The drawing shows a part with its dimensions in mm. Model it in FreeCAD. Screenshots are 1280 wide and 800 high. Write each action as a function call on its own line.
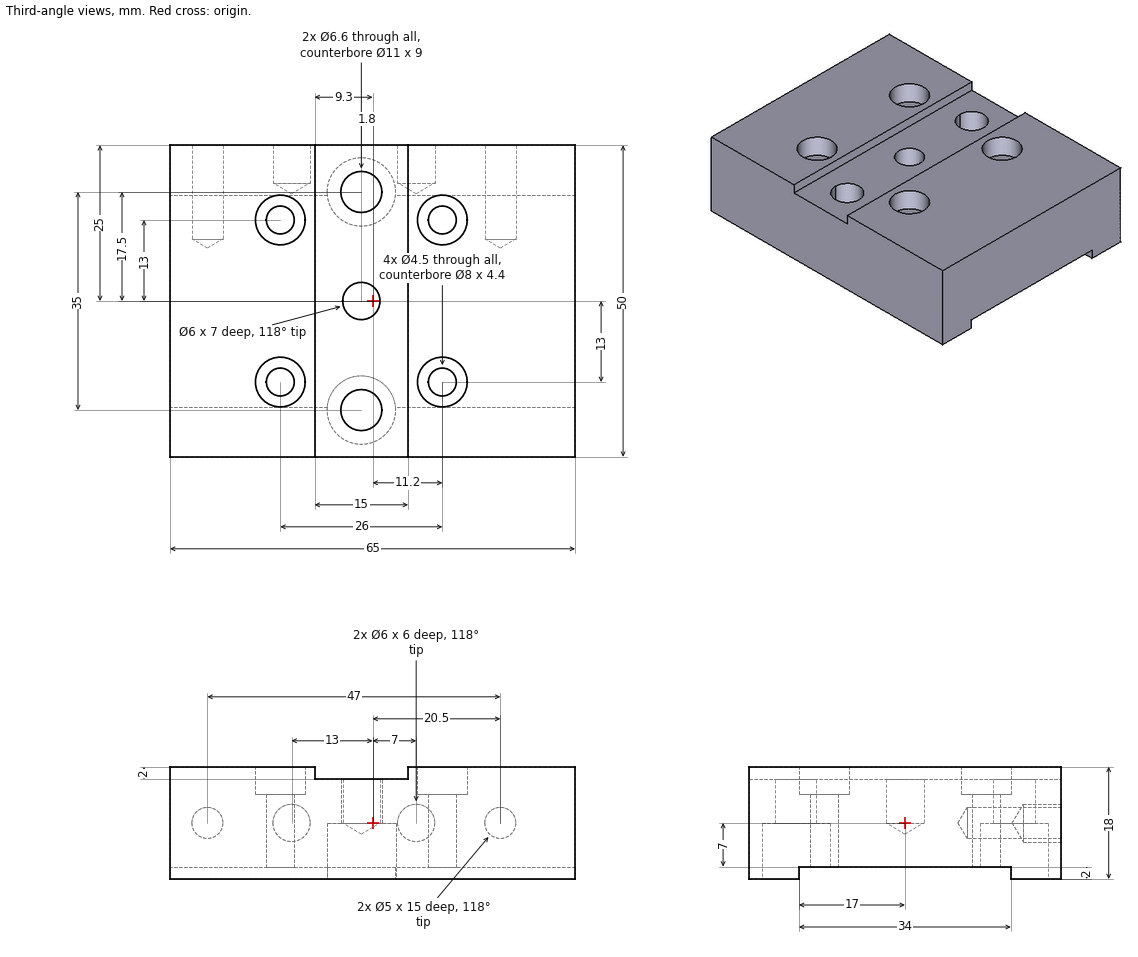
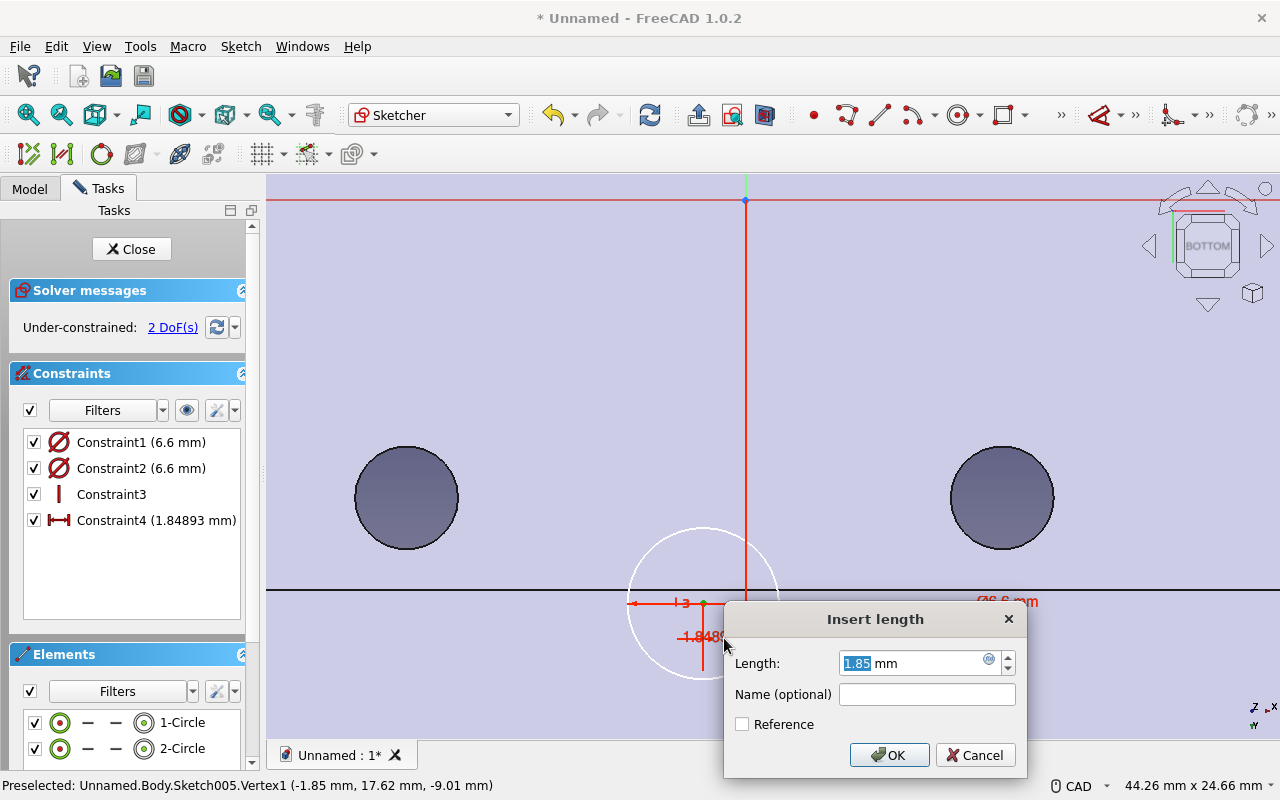
text(1.8)
key(Return)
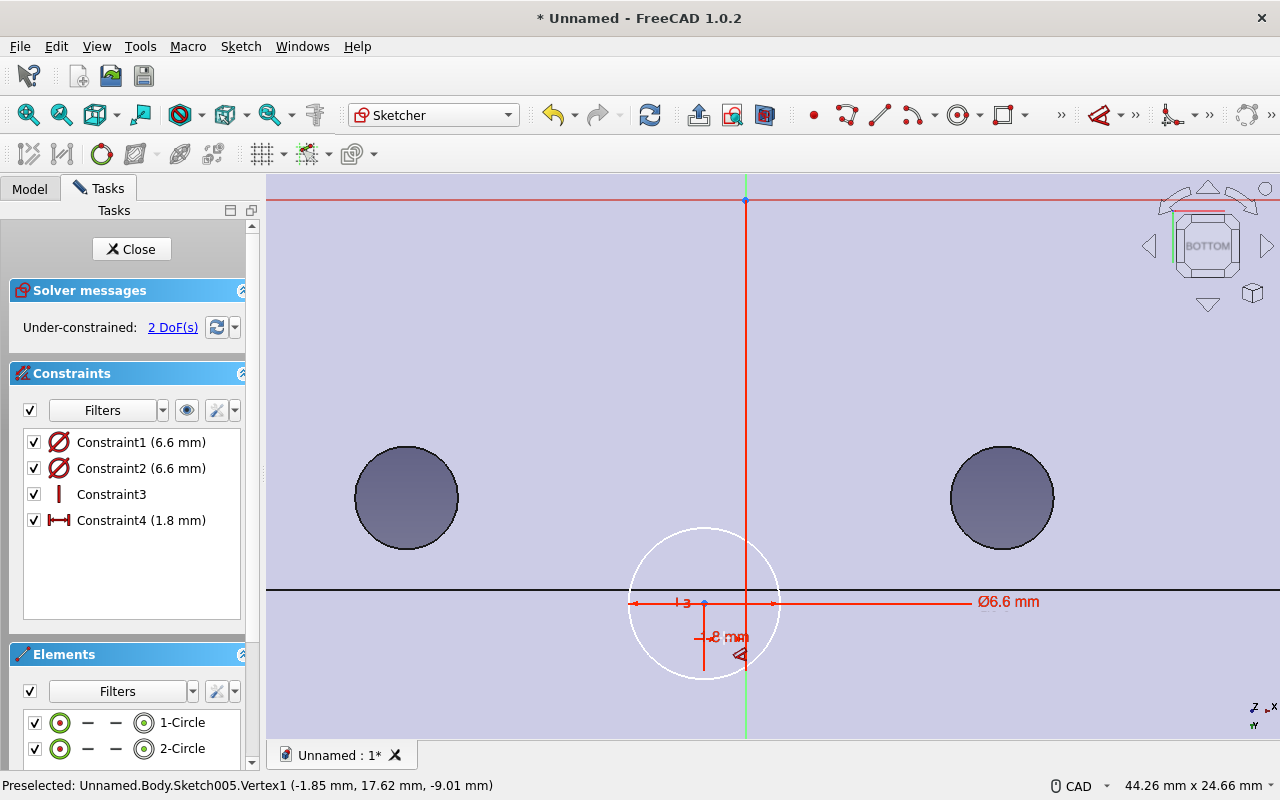
click(704, 604)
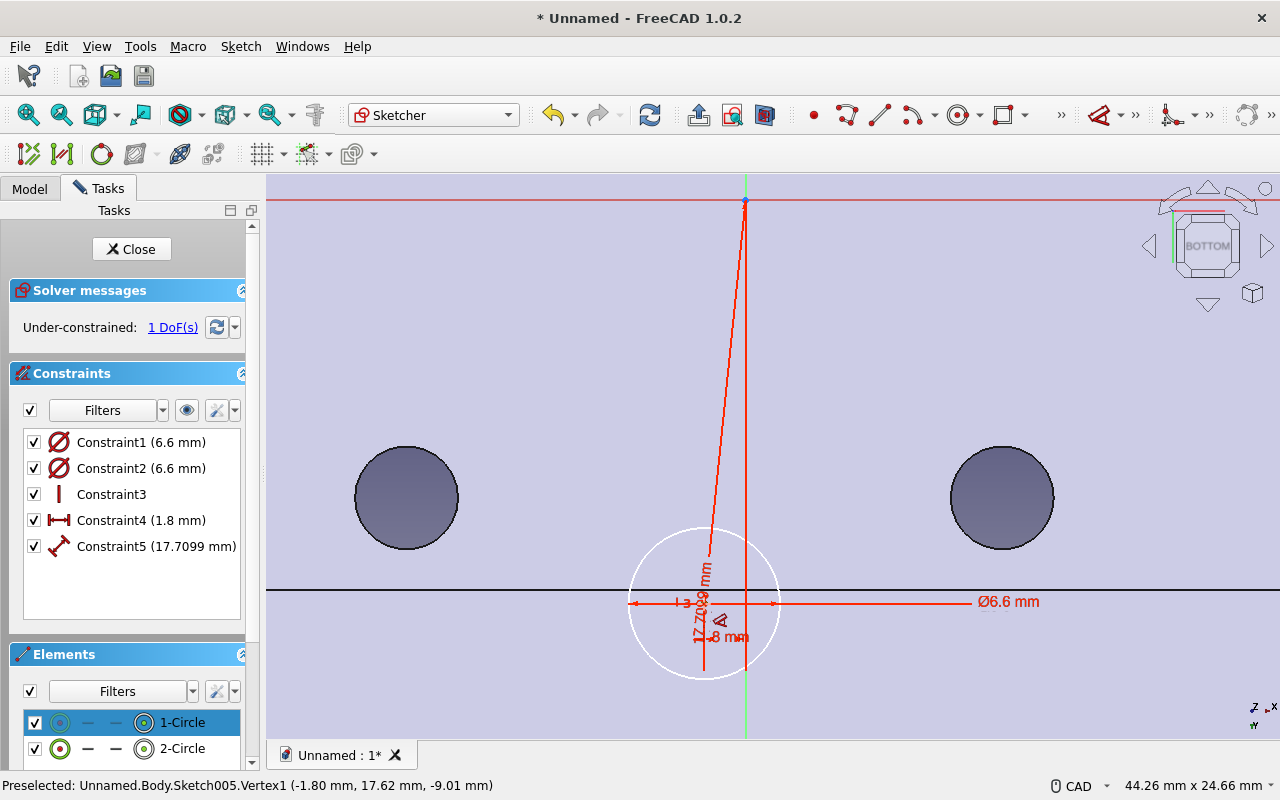
scroll(705, 606, down, 5)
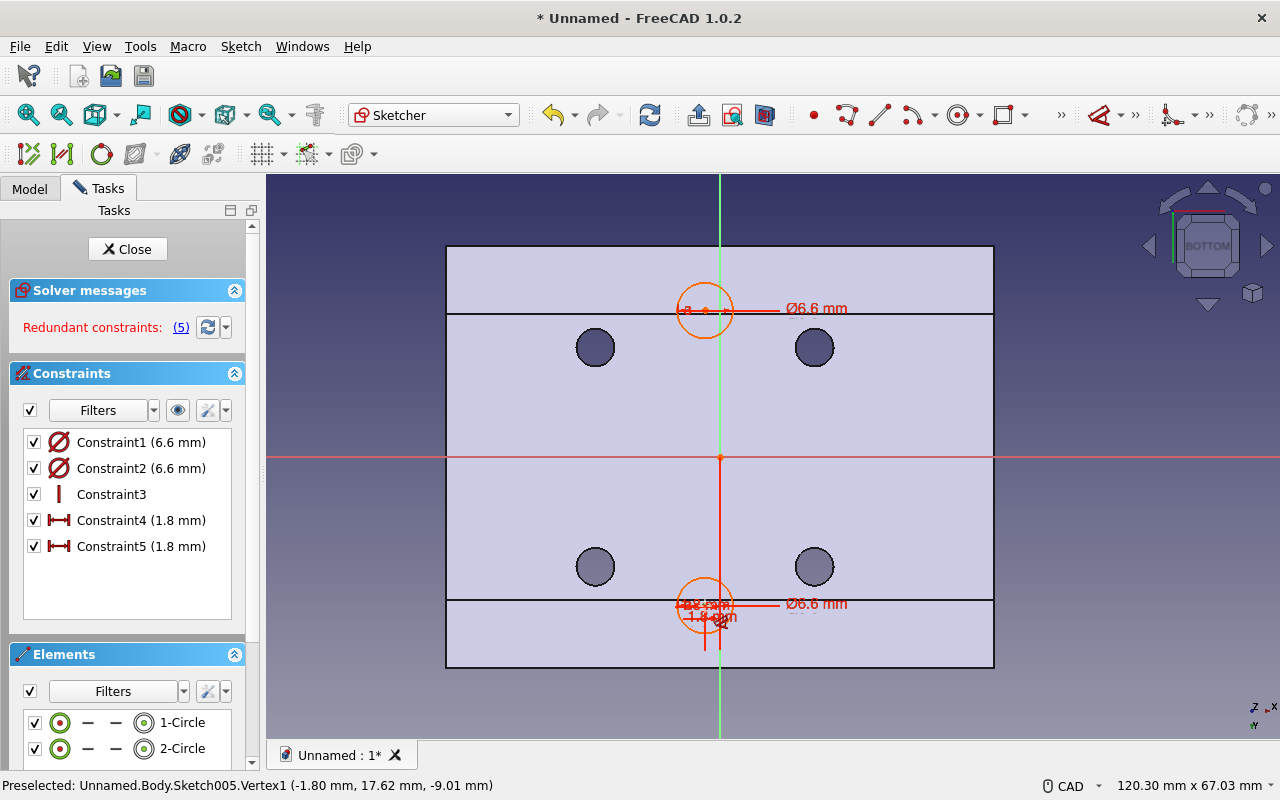
click(705, 311)
click(739, 390)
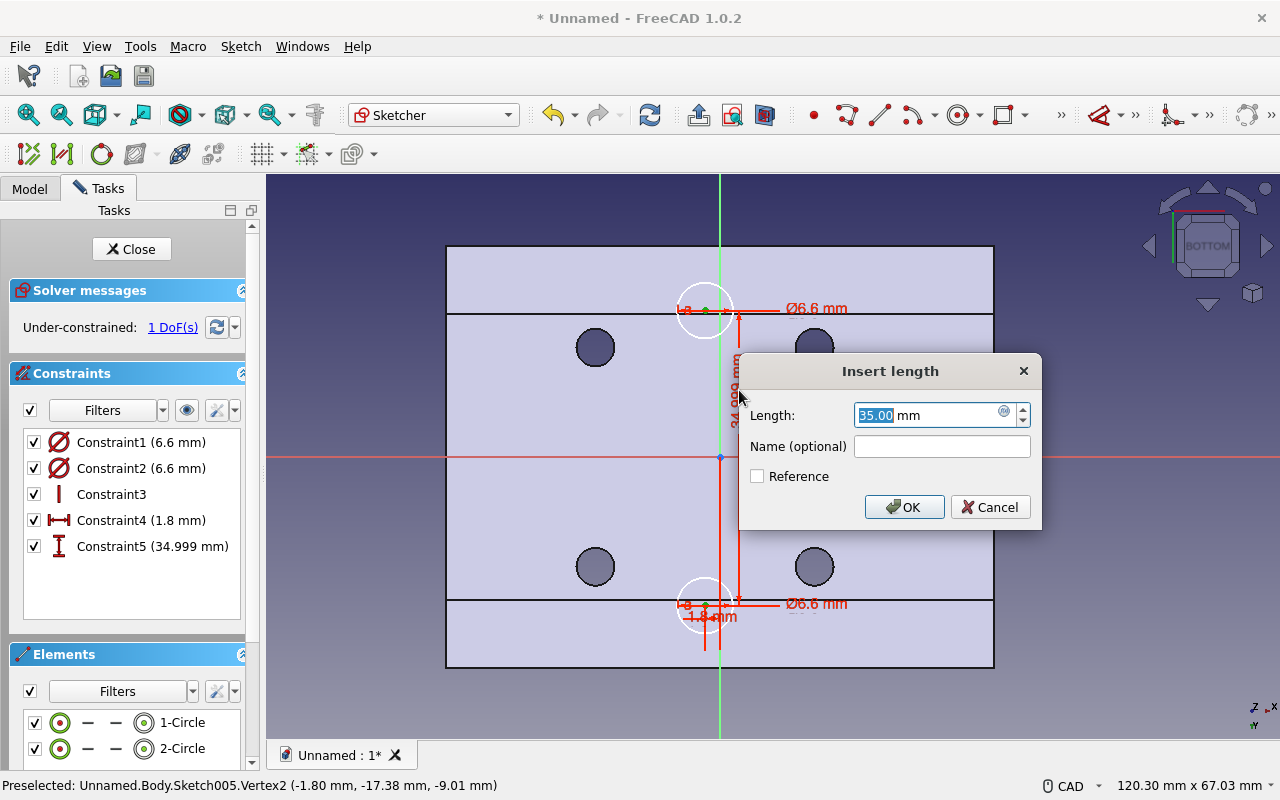
text(35)
key(Return)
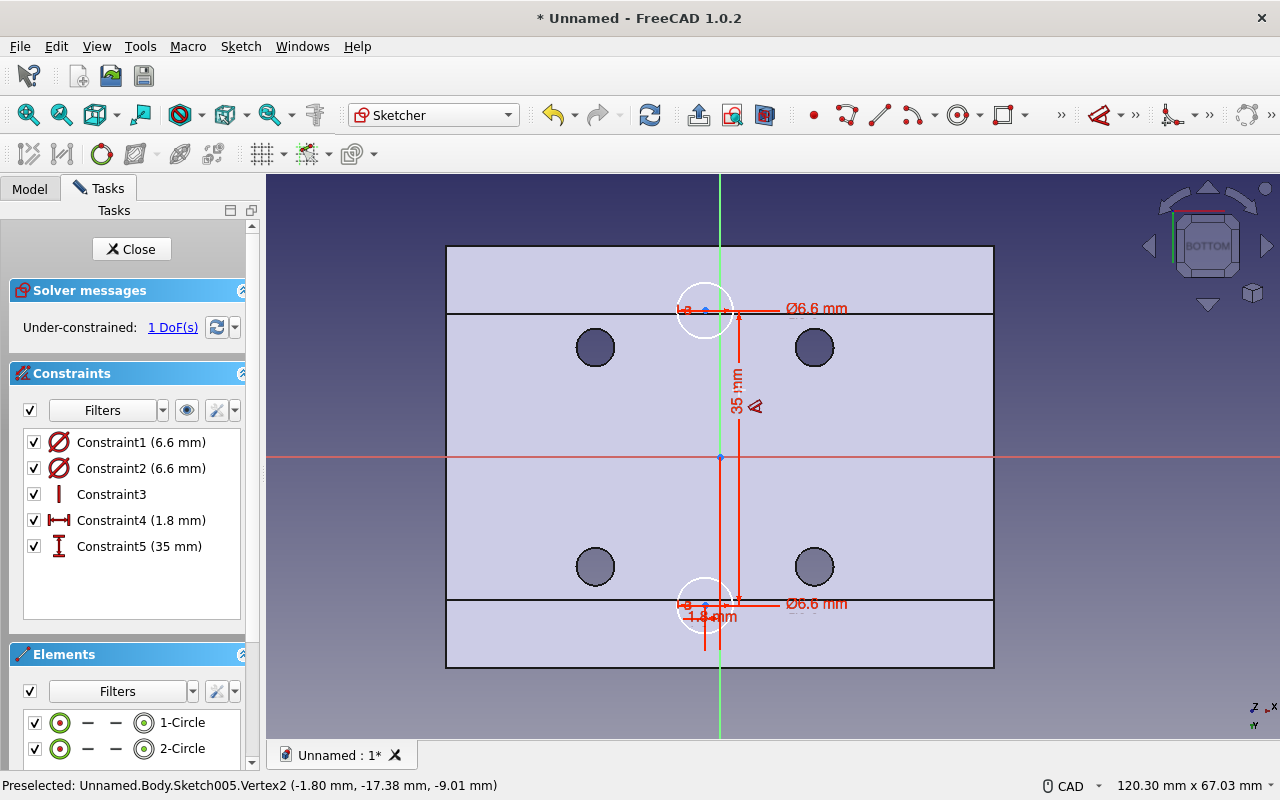
click(705, 606)
click(754, 531)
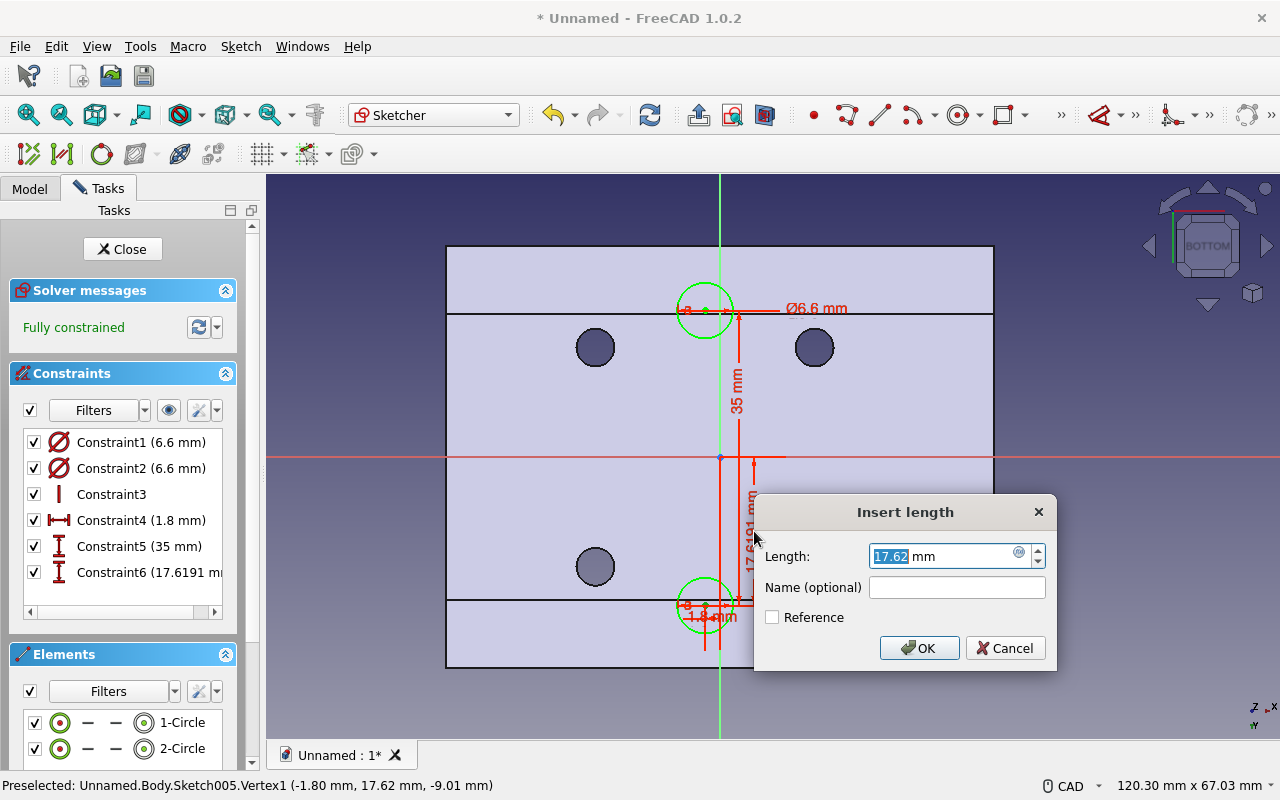
text(17.5)
key(Return)
key(Escape)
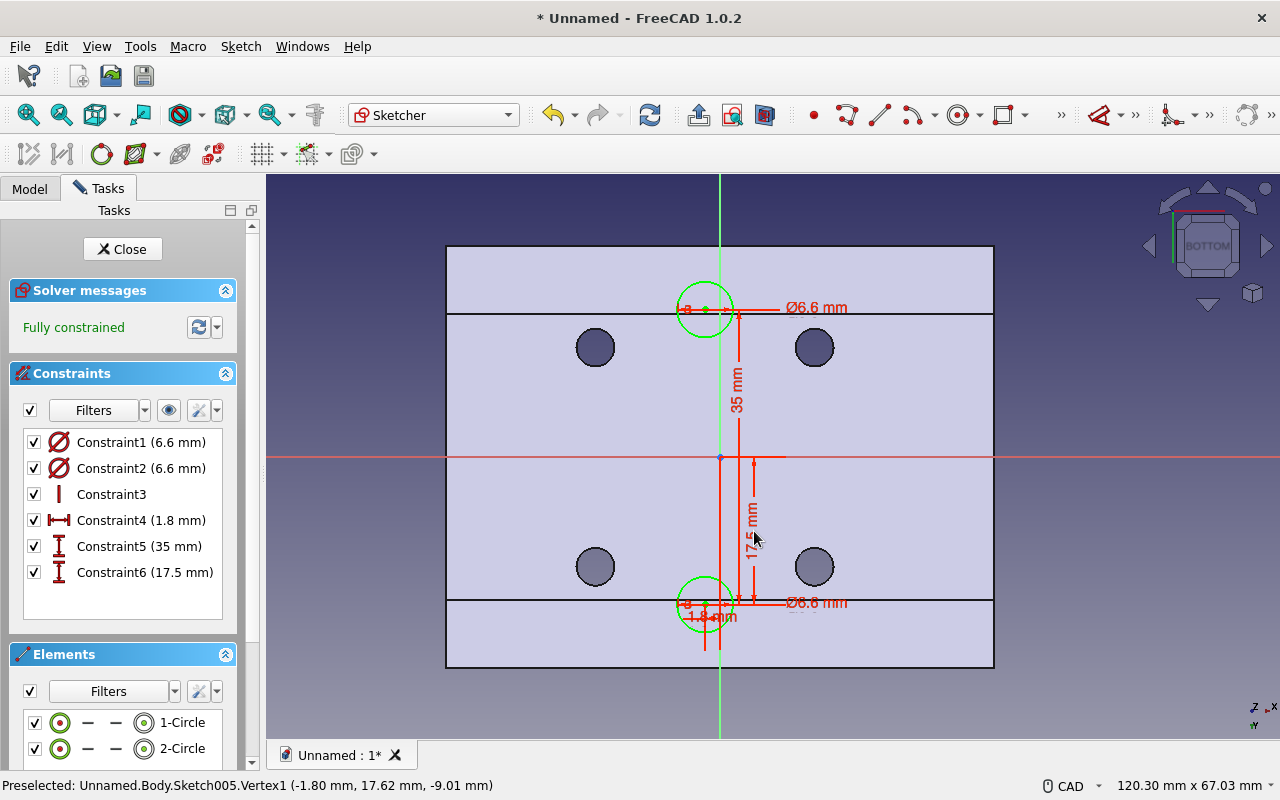
click(123, 249)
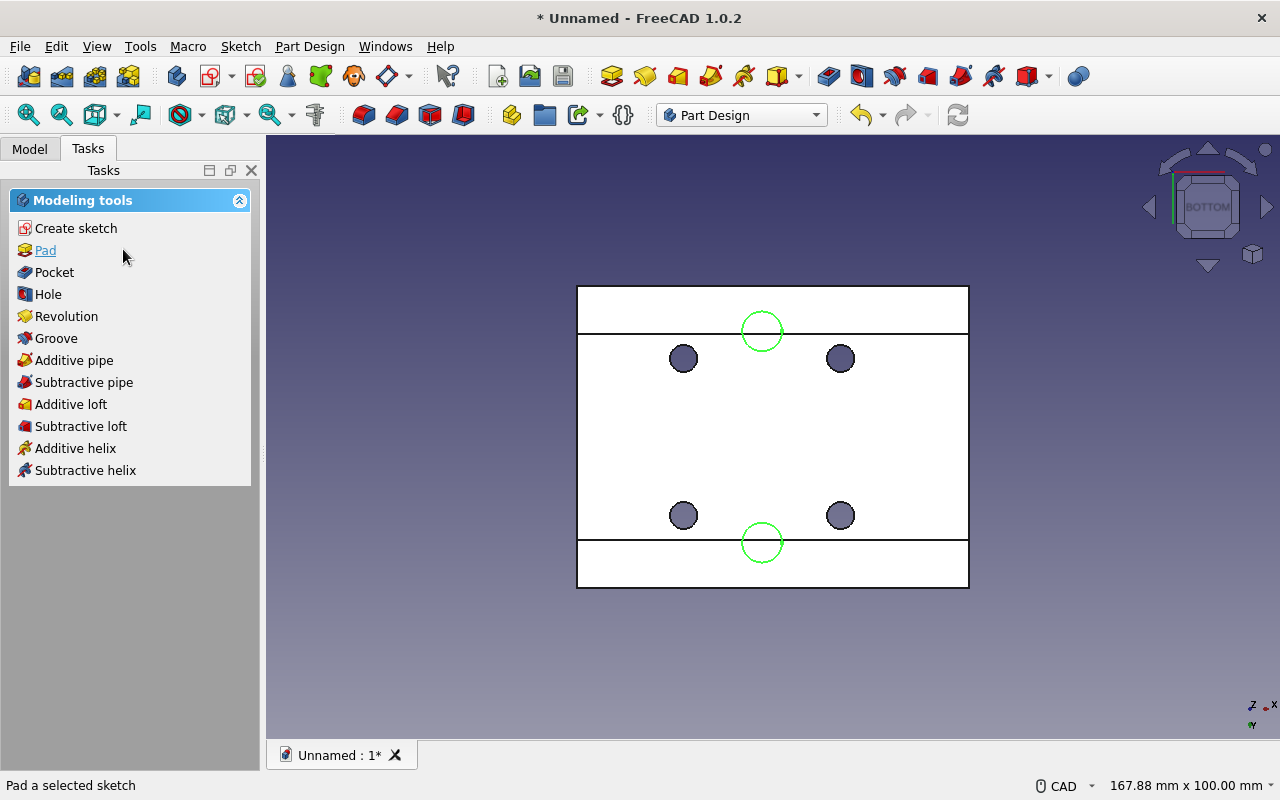
click(862, 76)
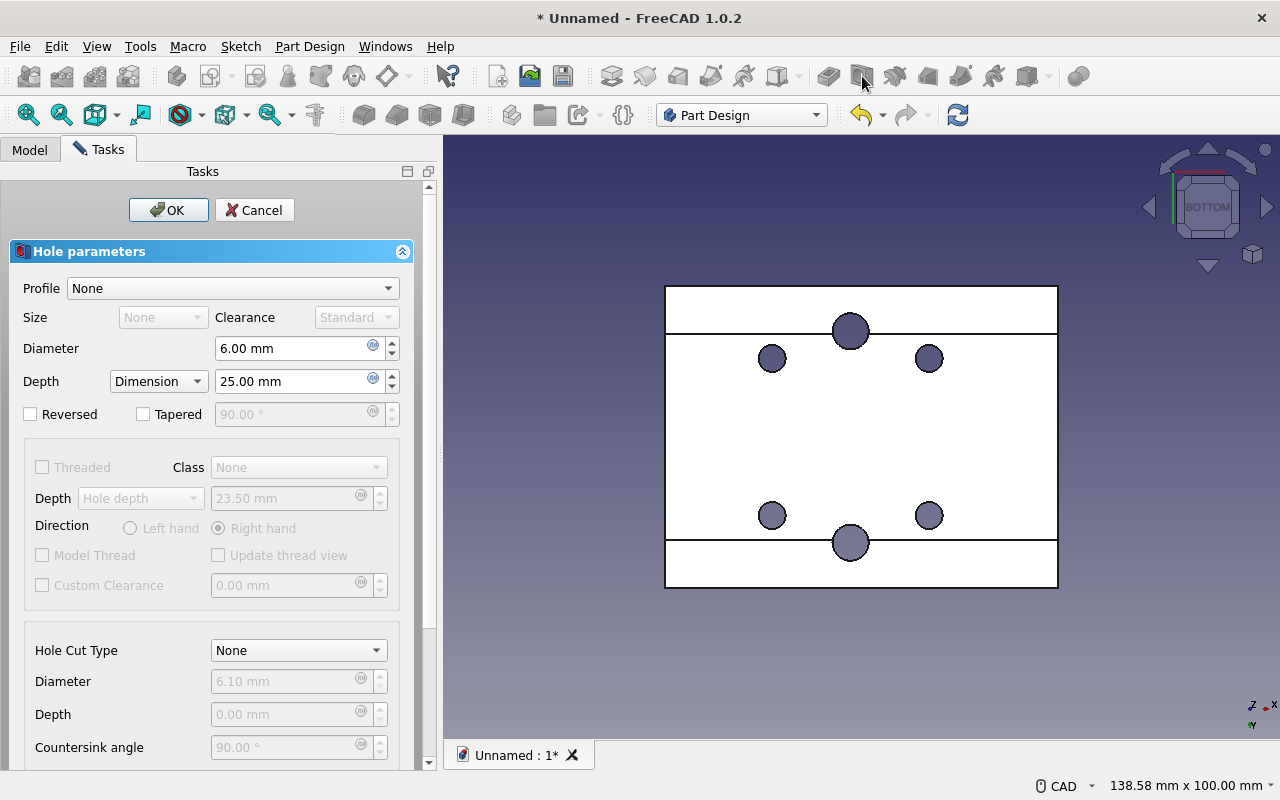
triple_click(300, 348)